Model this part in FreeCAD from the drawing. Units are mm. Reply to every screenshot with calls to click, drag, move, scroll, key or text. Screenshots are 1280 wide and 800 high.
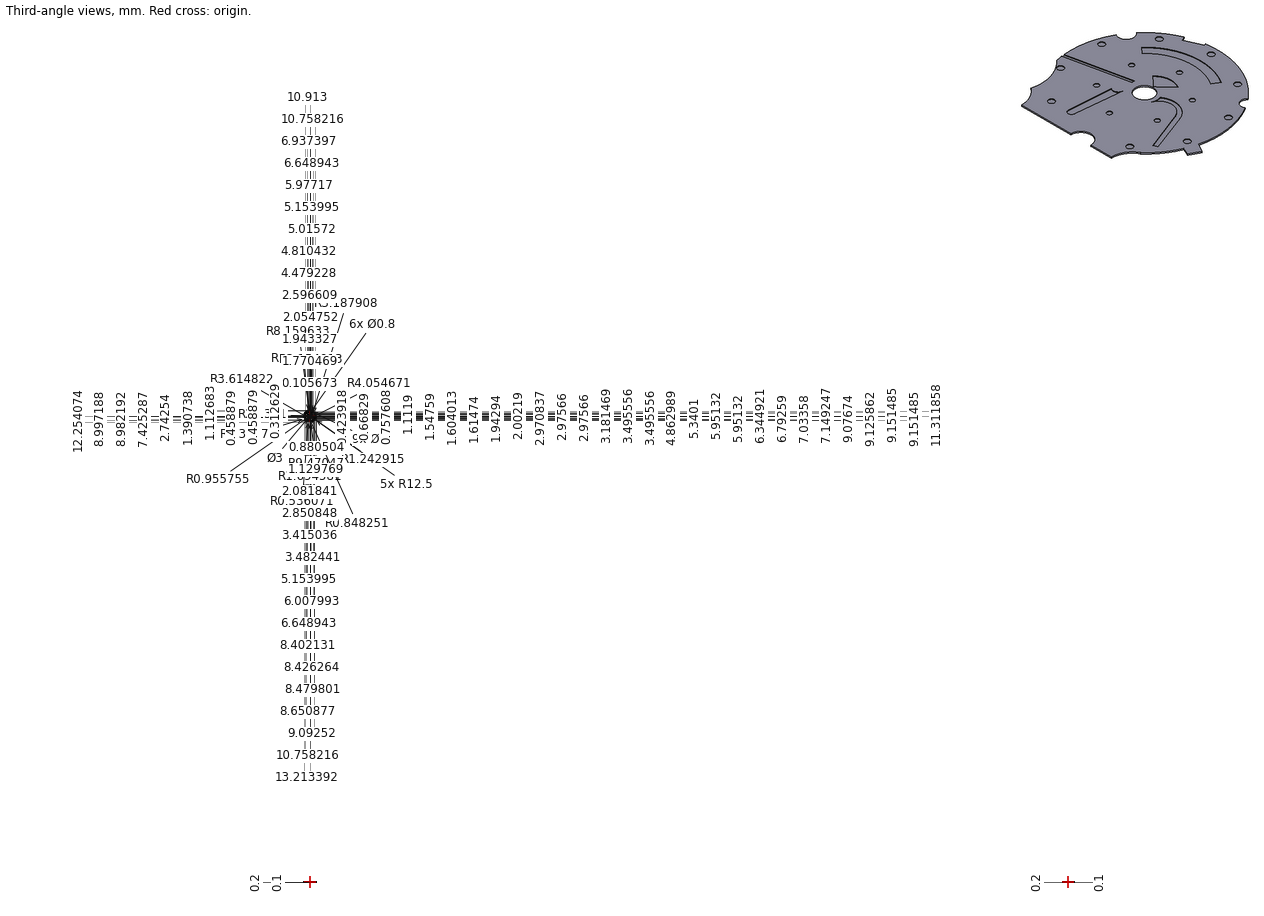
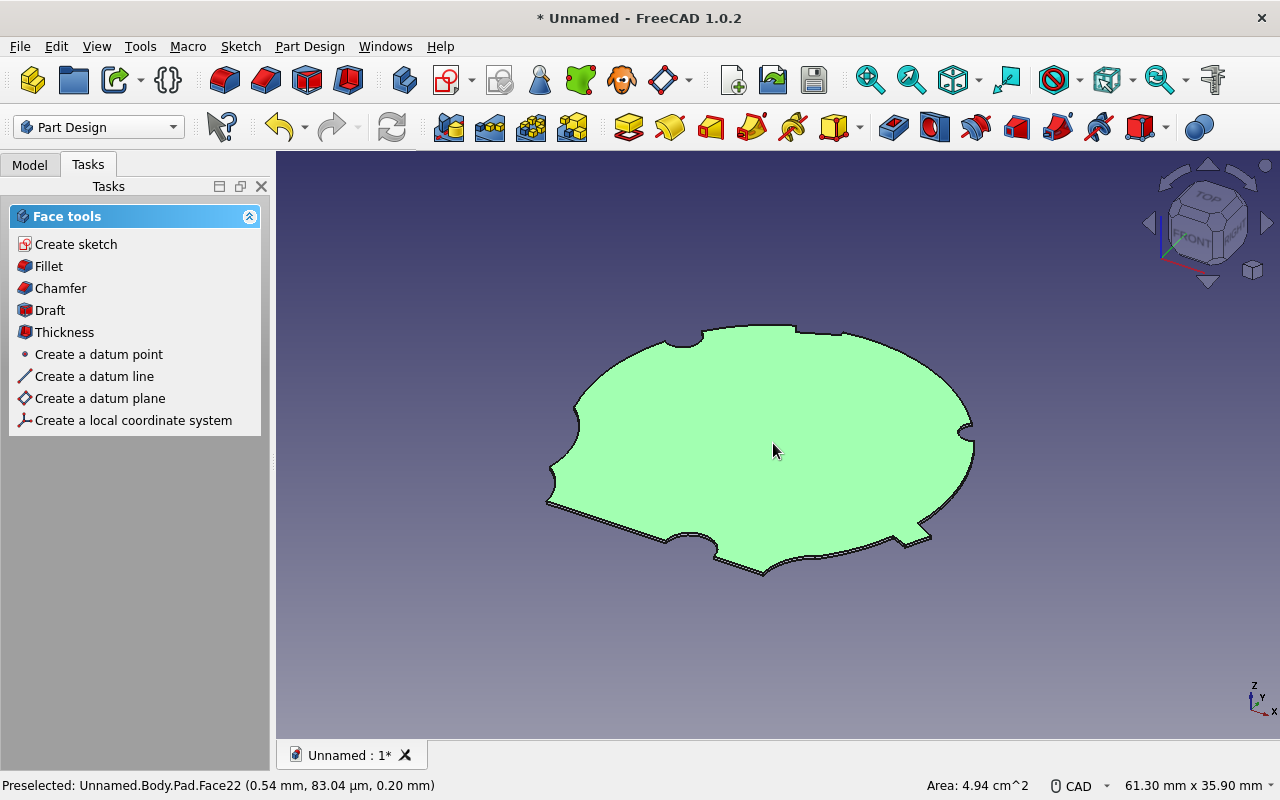
click(446, 80)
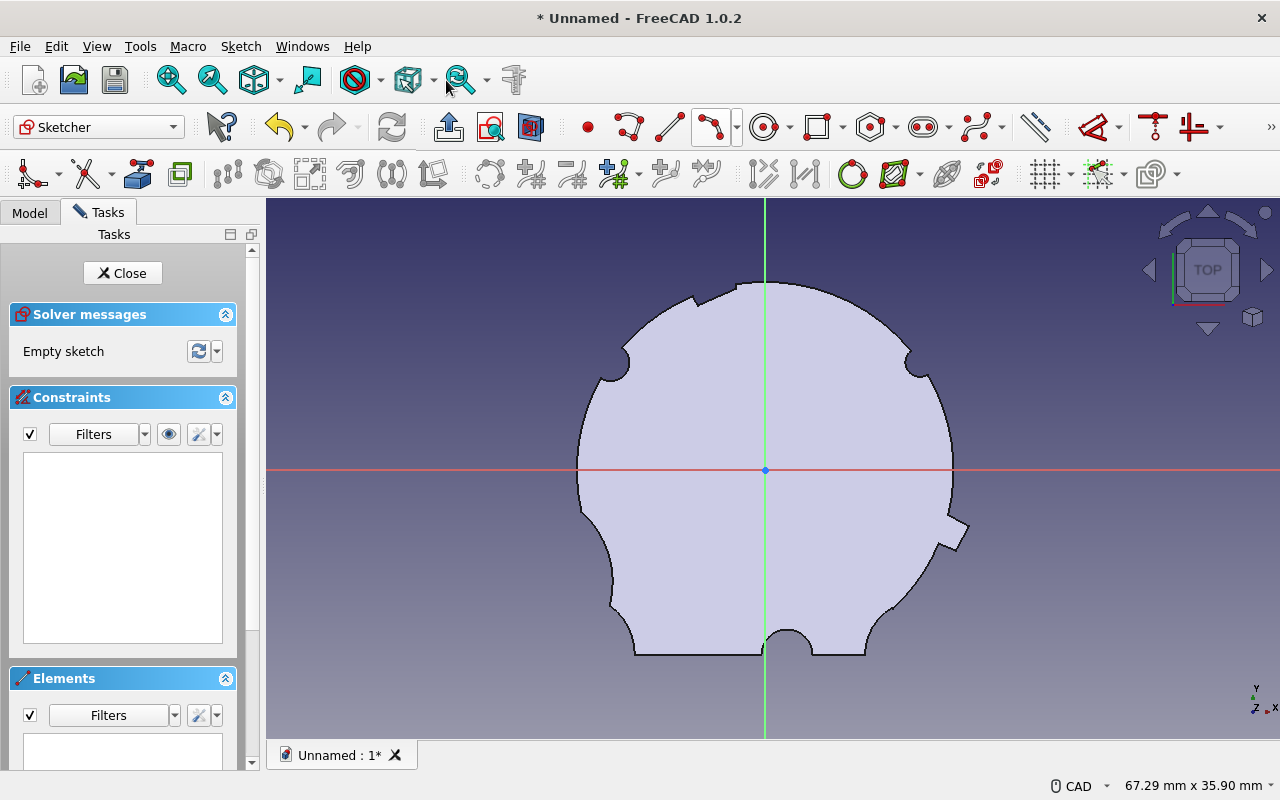
scroll(775, 470, up, 10)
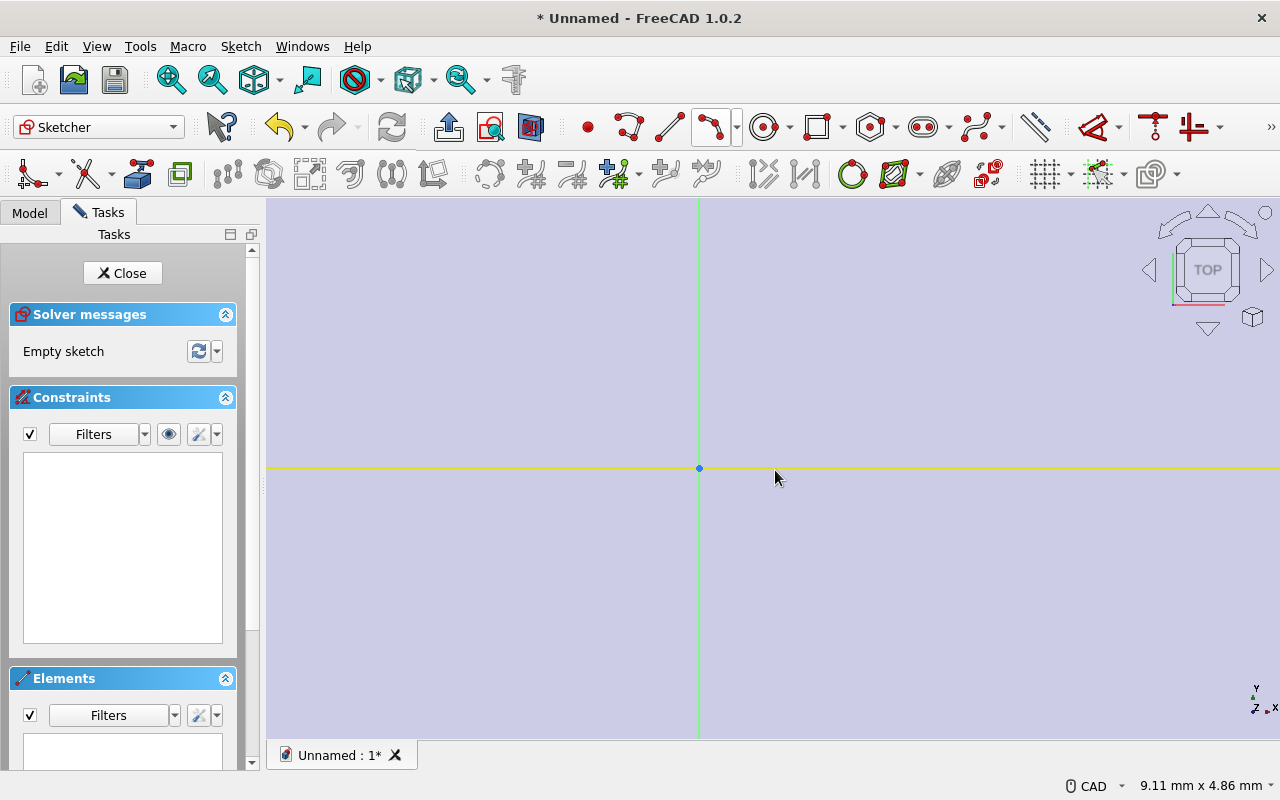
click(764, 128)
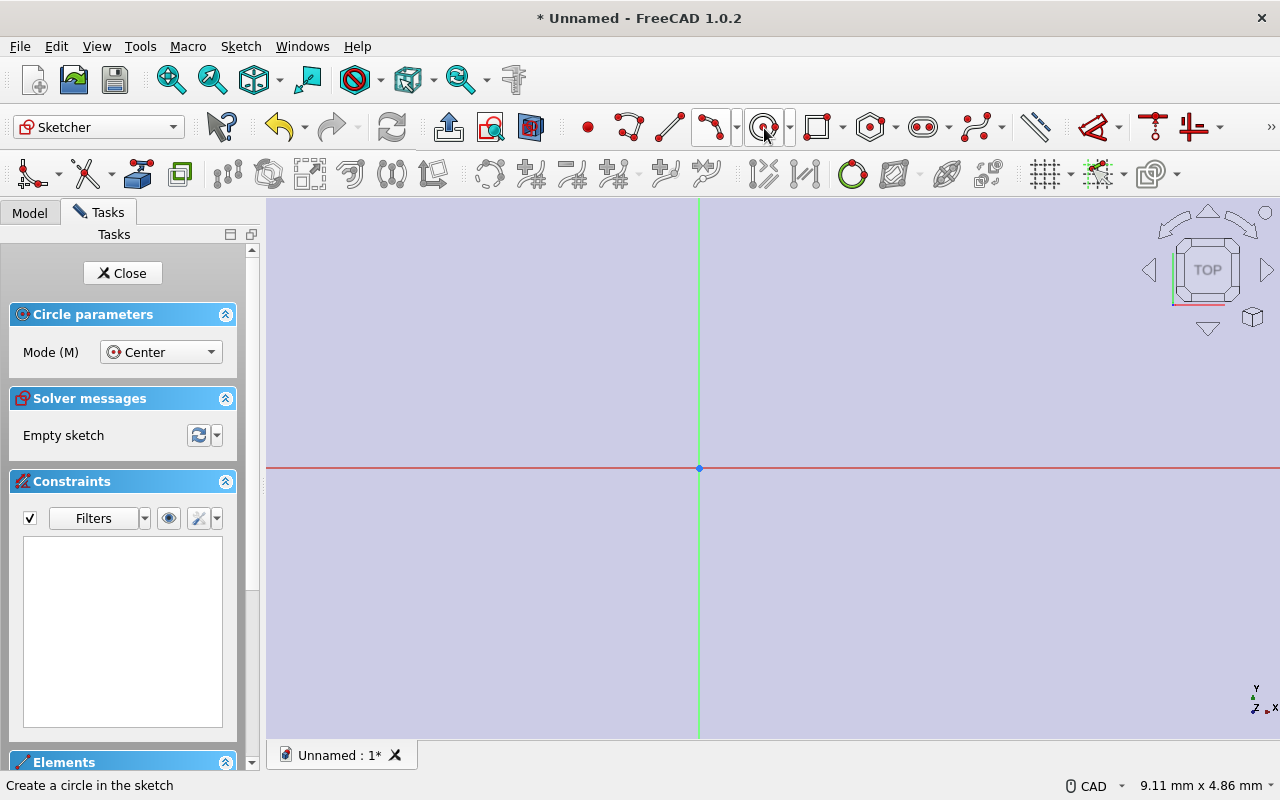
click(699, 468)
click(818, 350)
key(Escape)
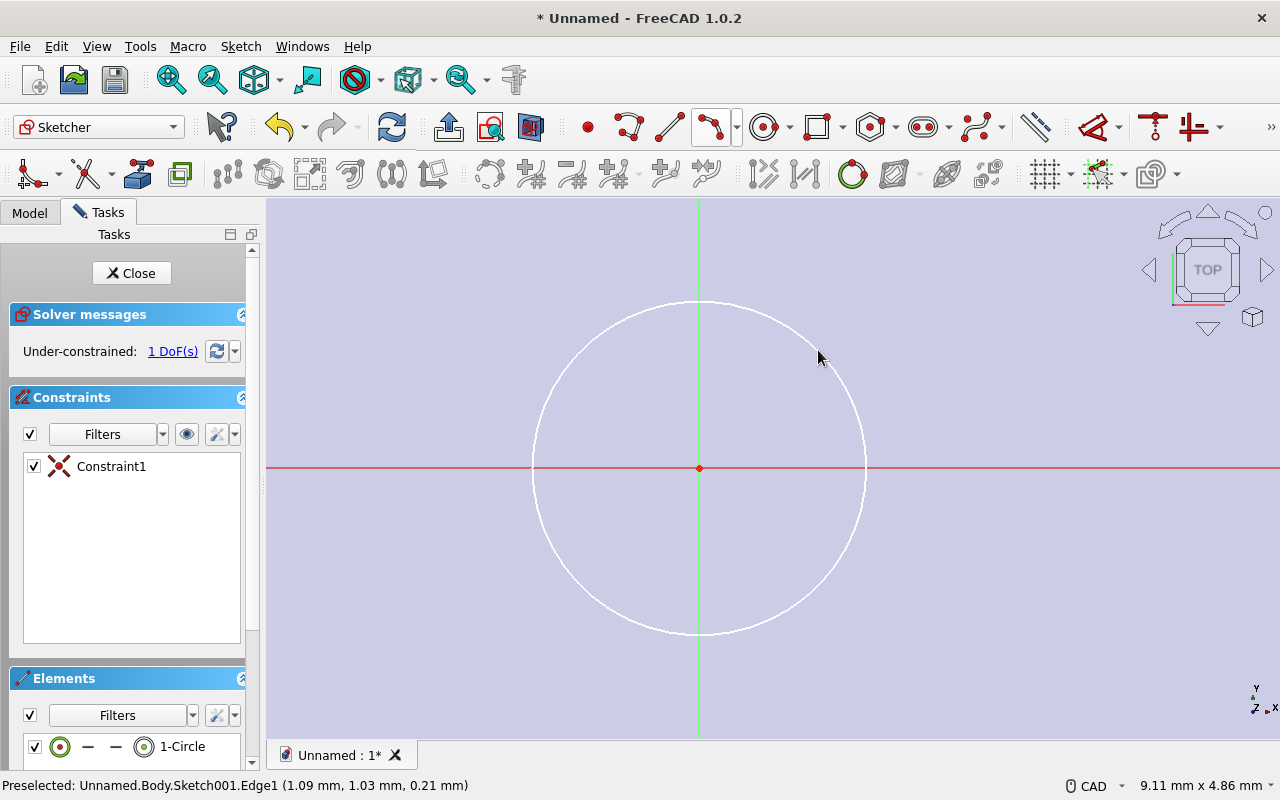
click(1092, 128)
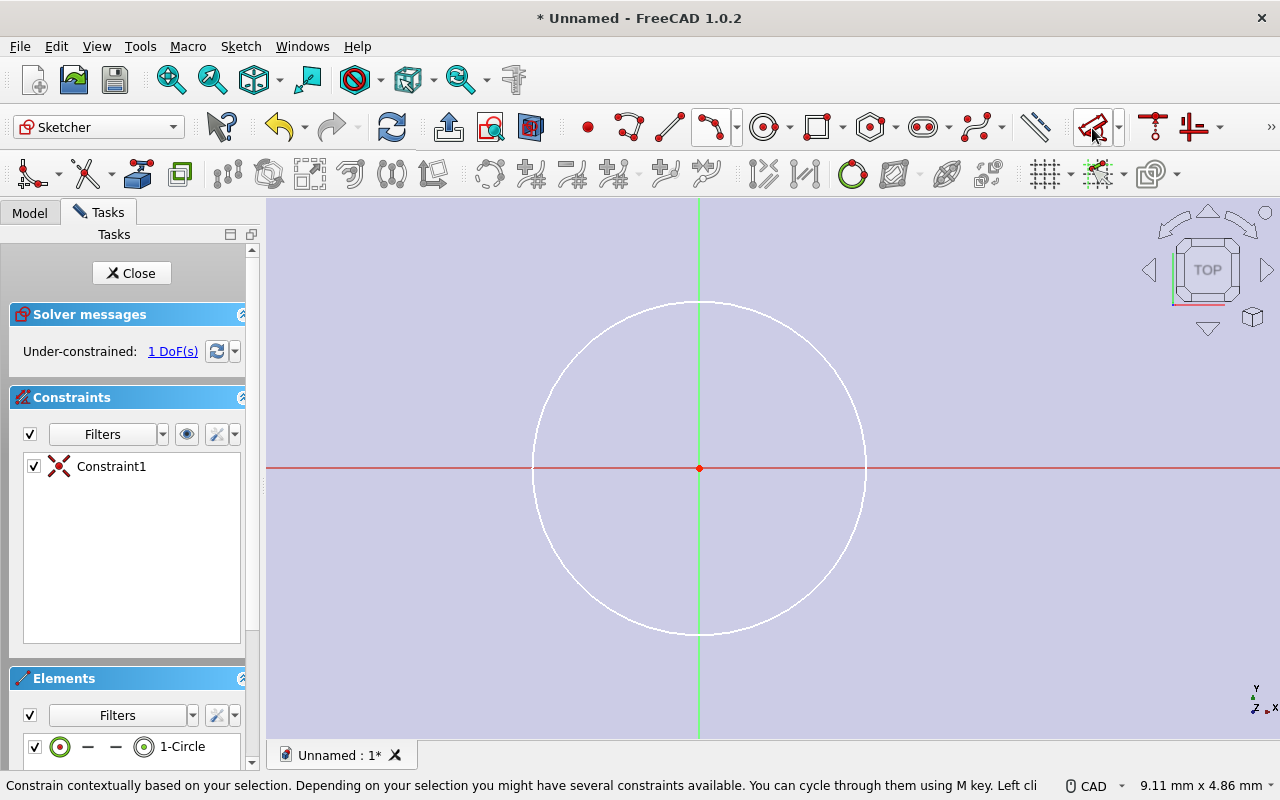
click(817, 350)
click(840, 327)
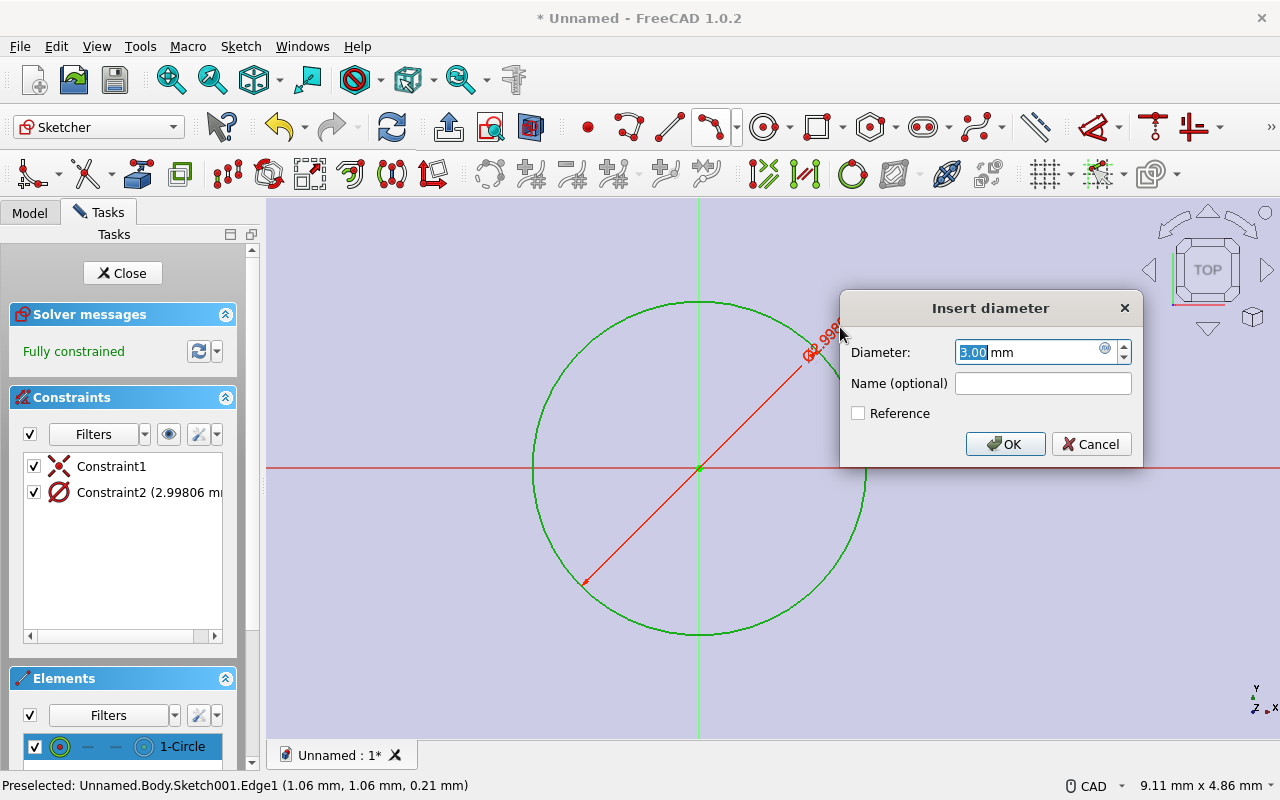
text(3)
key(Return)
key(Escape)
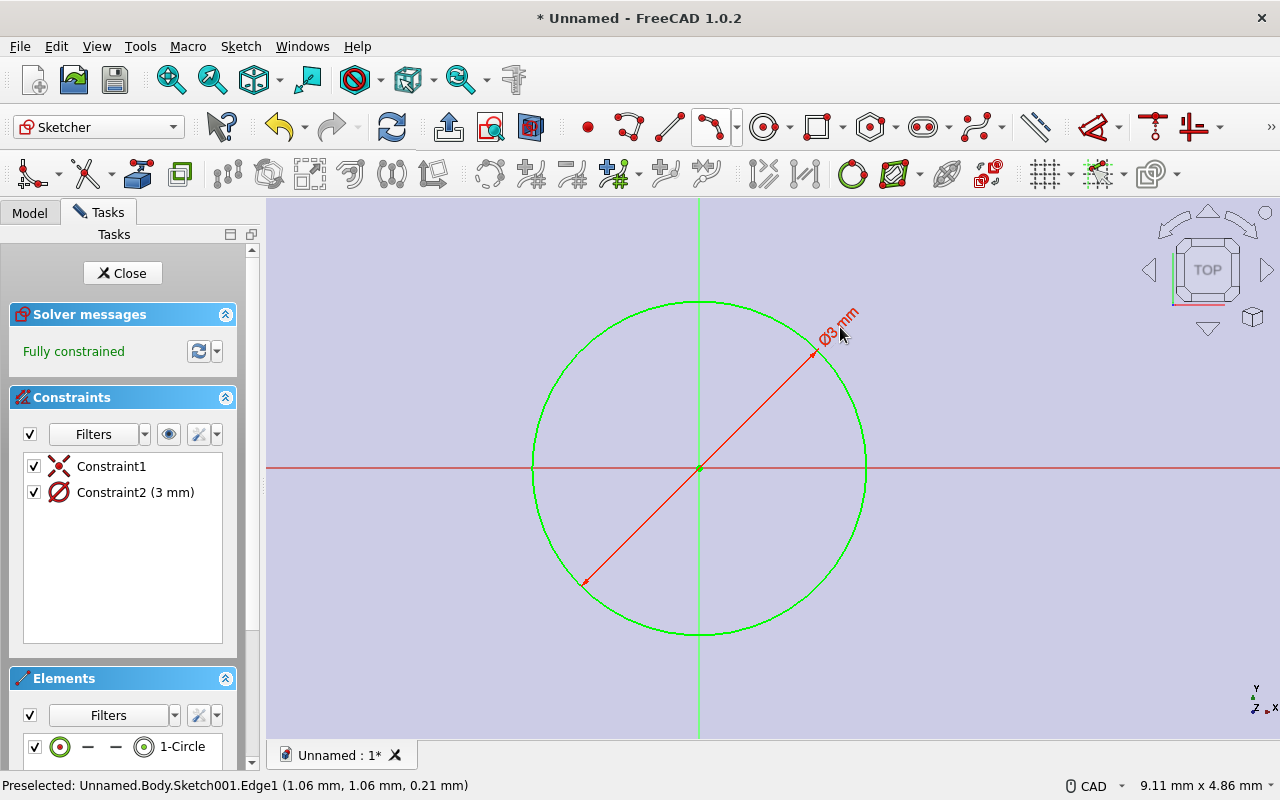
click(123, 273)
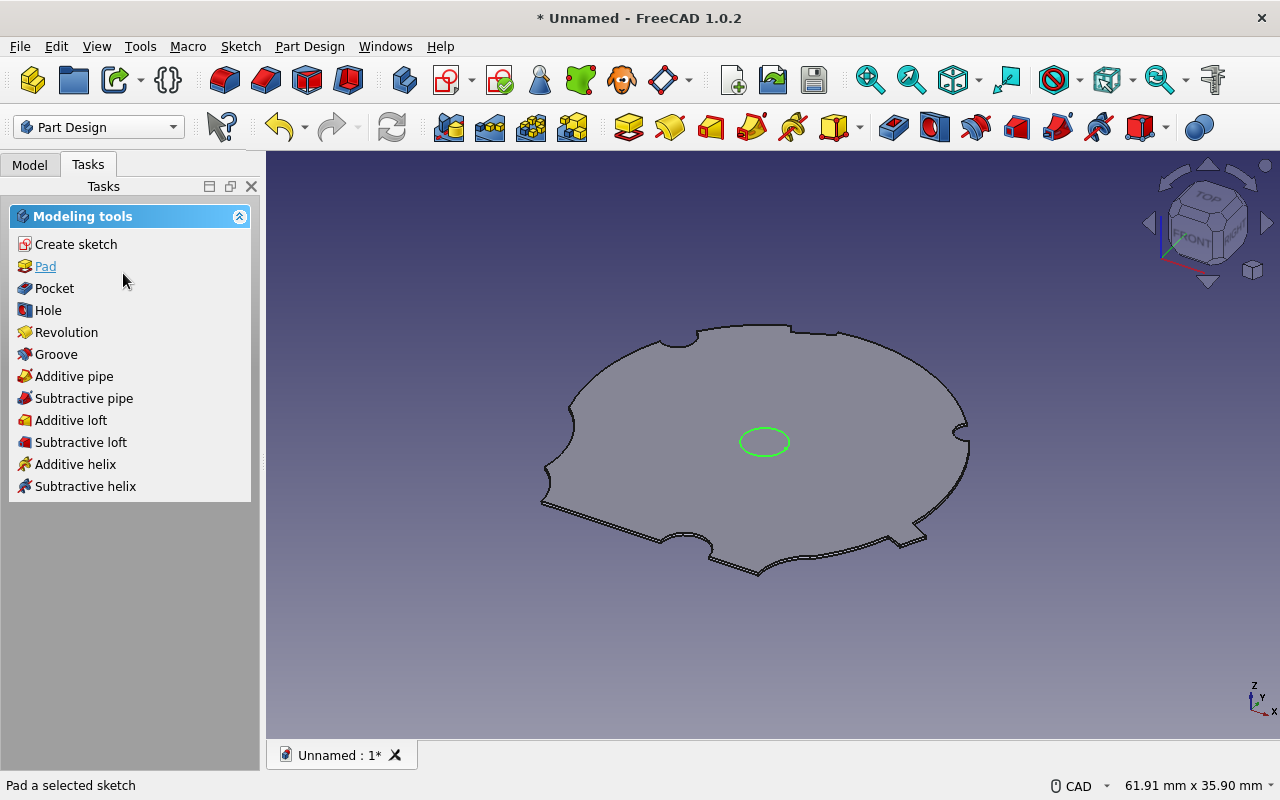
click(894, 128)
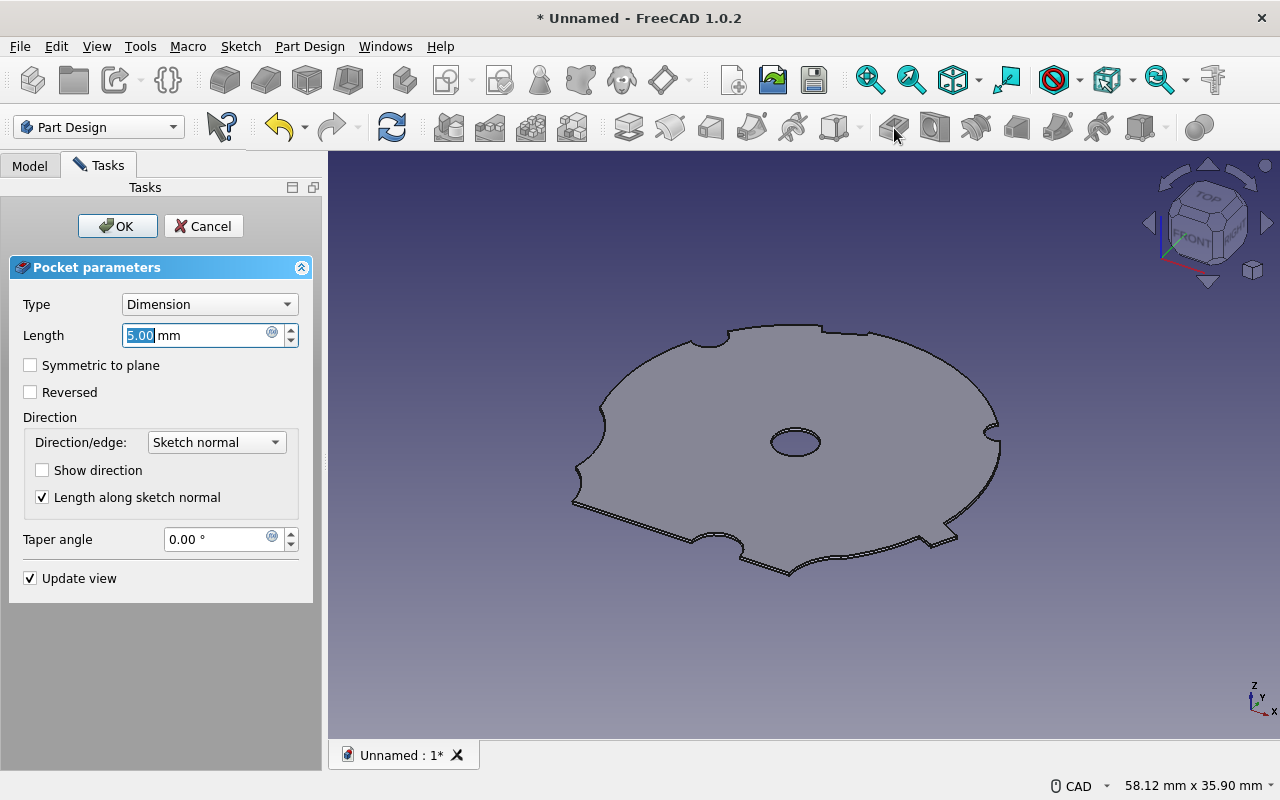
text(0.2)
key(Tab)